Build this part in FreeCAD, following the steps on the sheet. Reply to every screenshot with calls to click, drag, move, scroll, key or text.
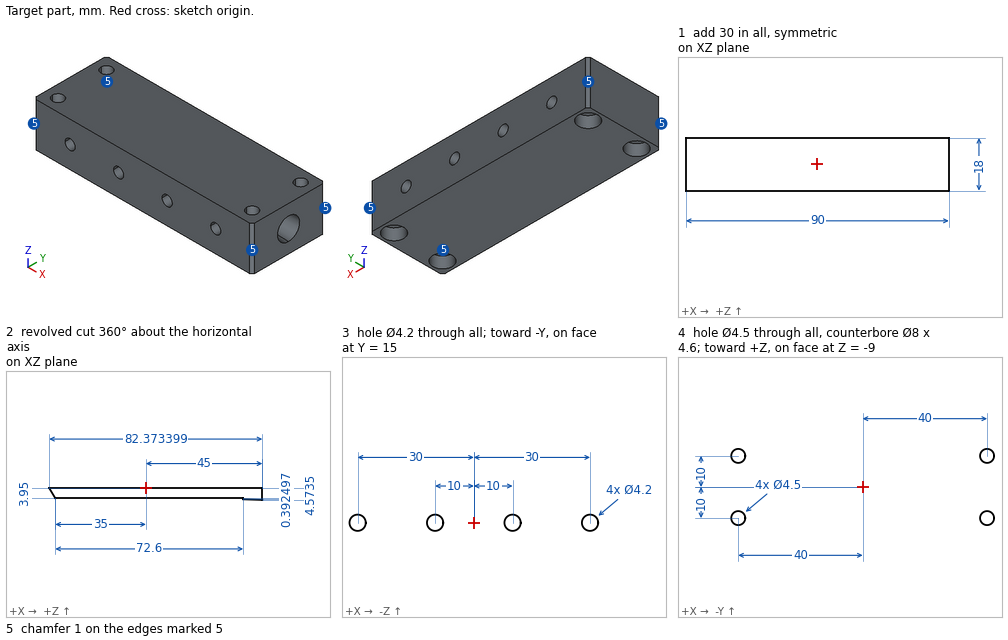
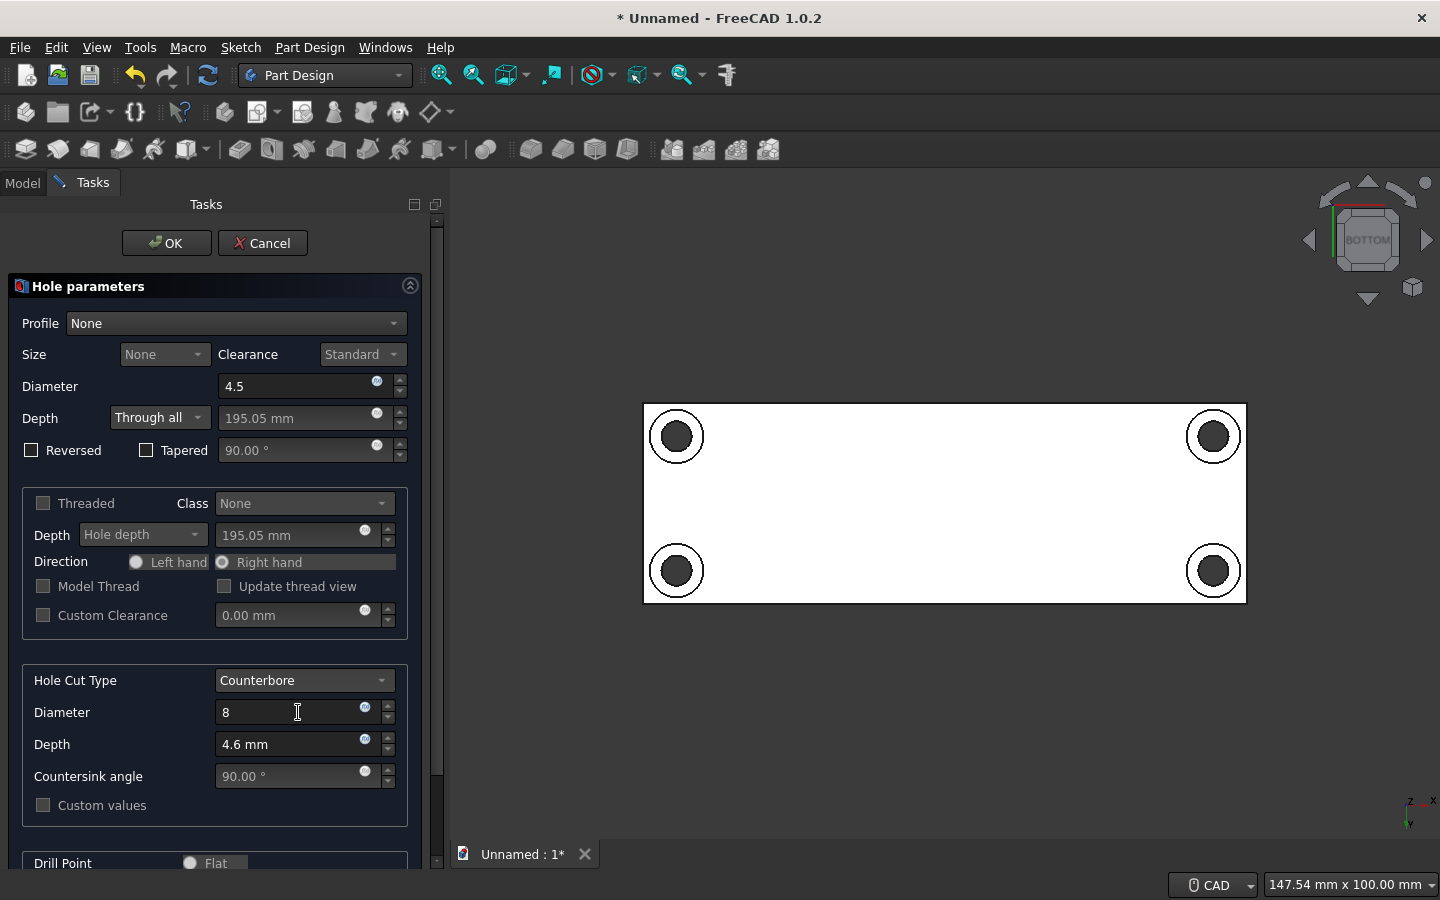
click(167, 243)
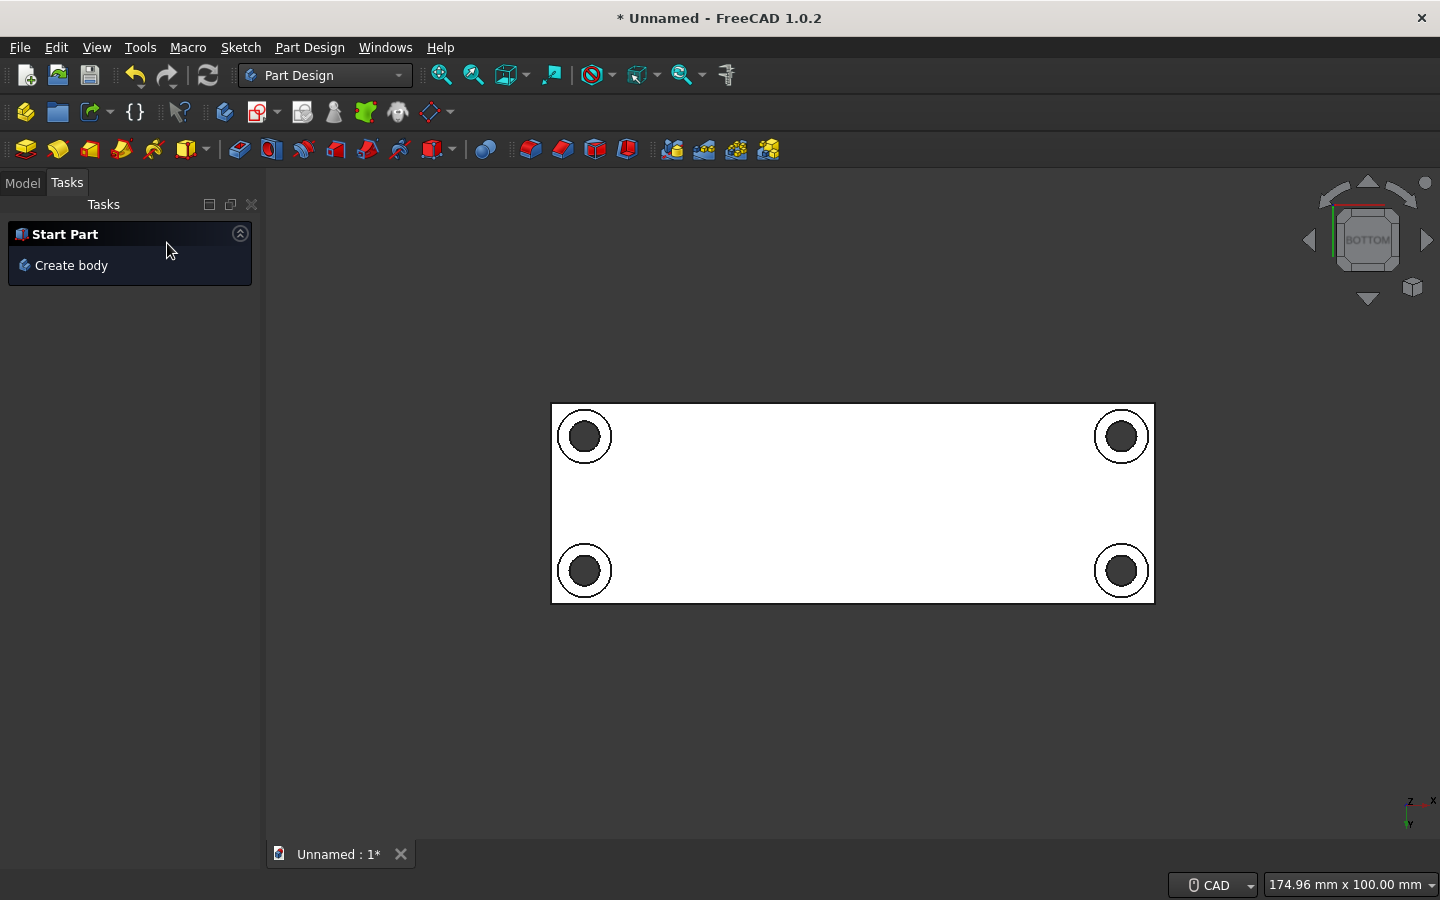
key(0)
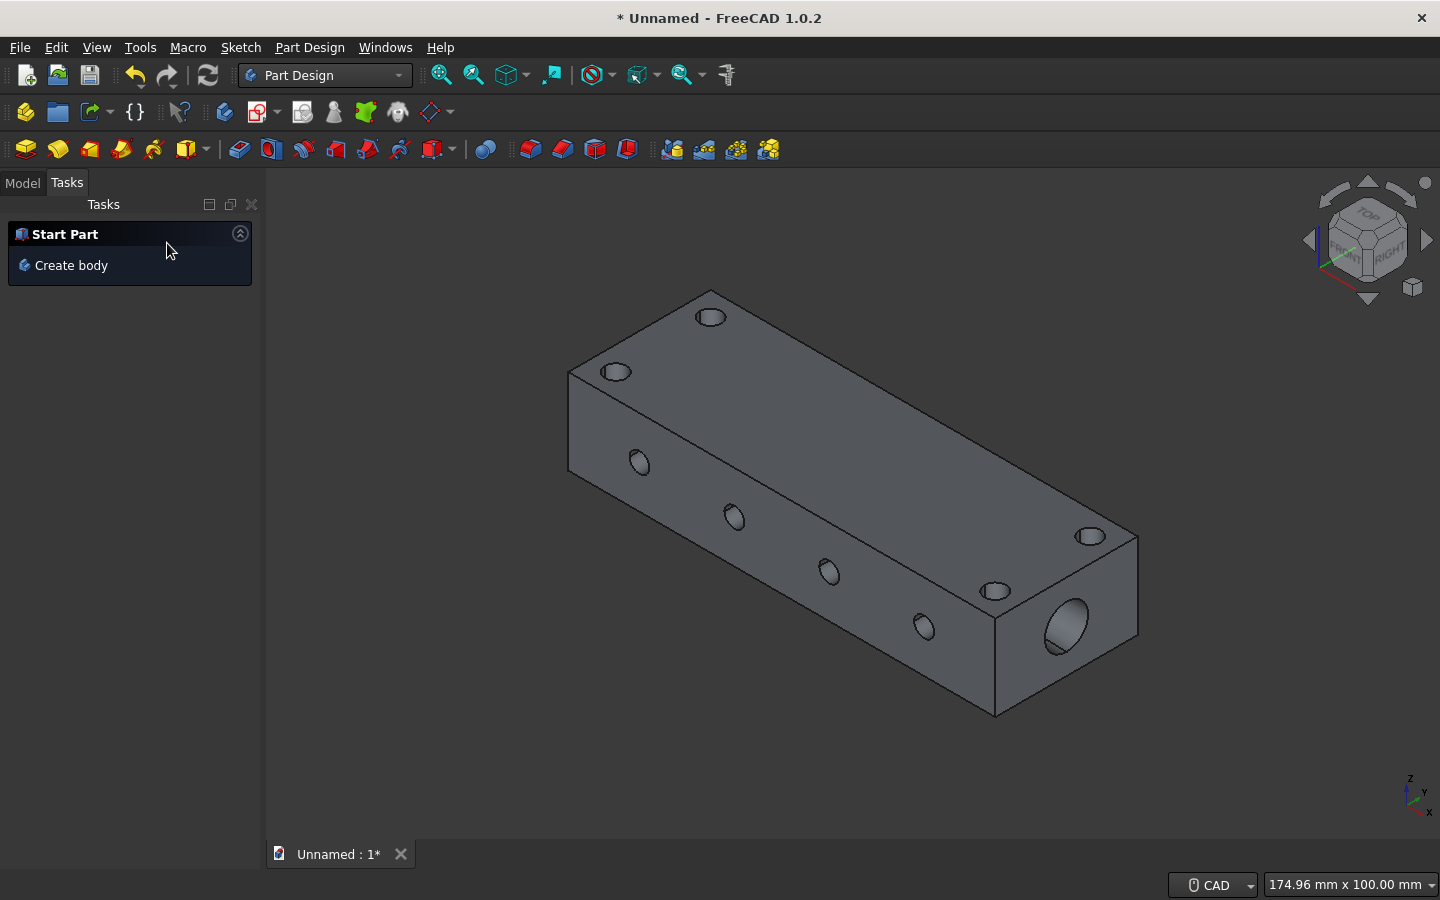
click(995, 667)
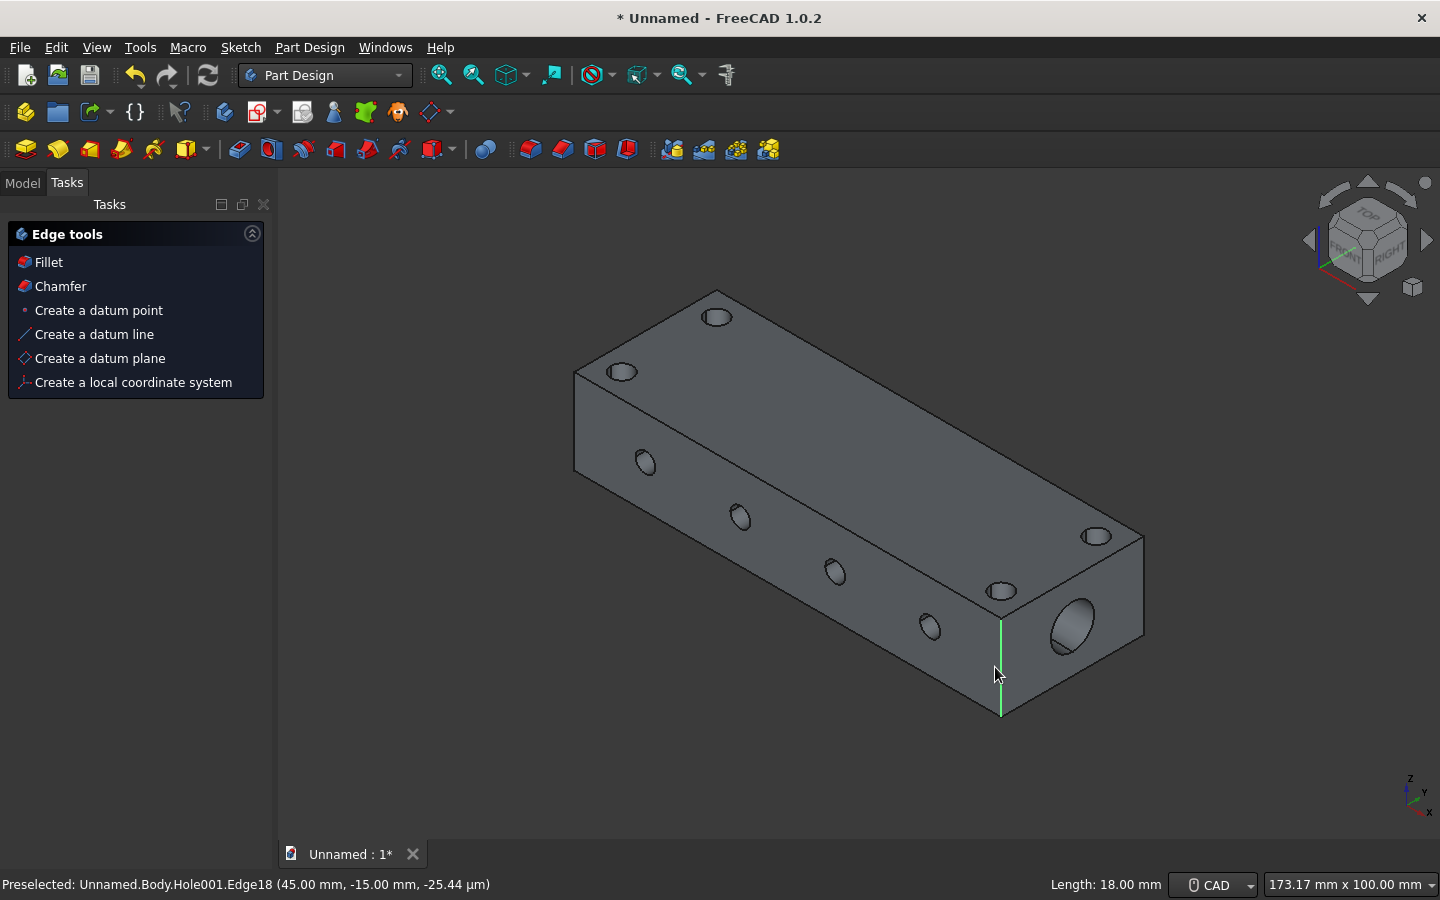
key(2)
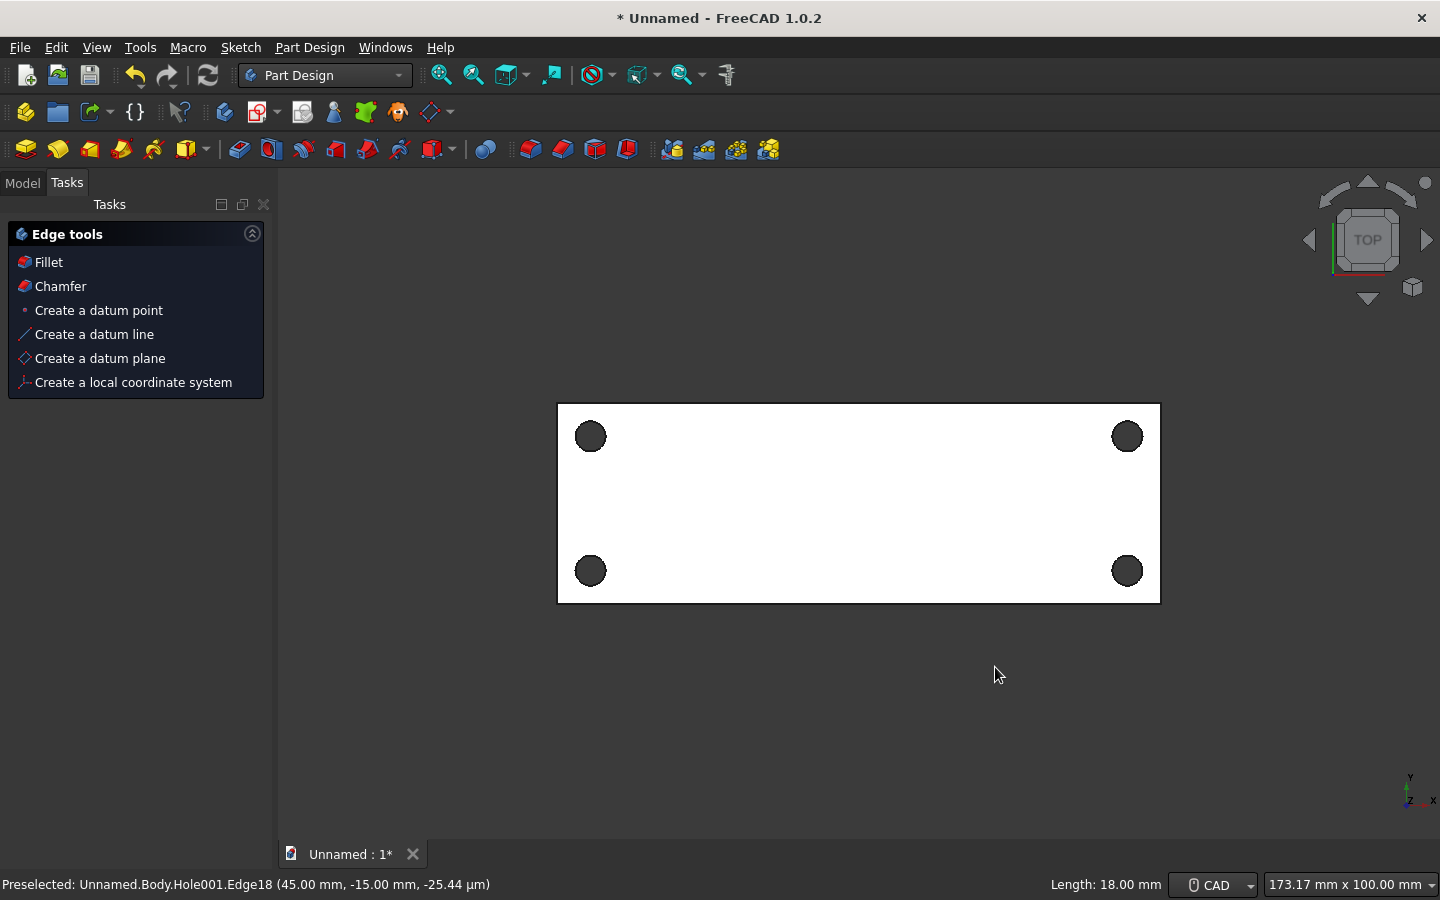
key(1)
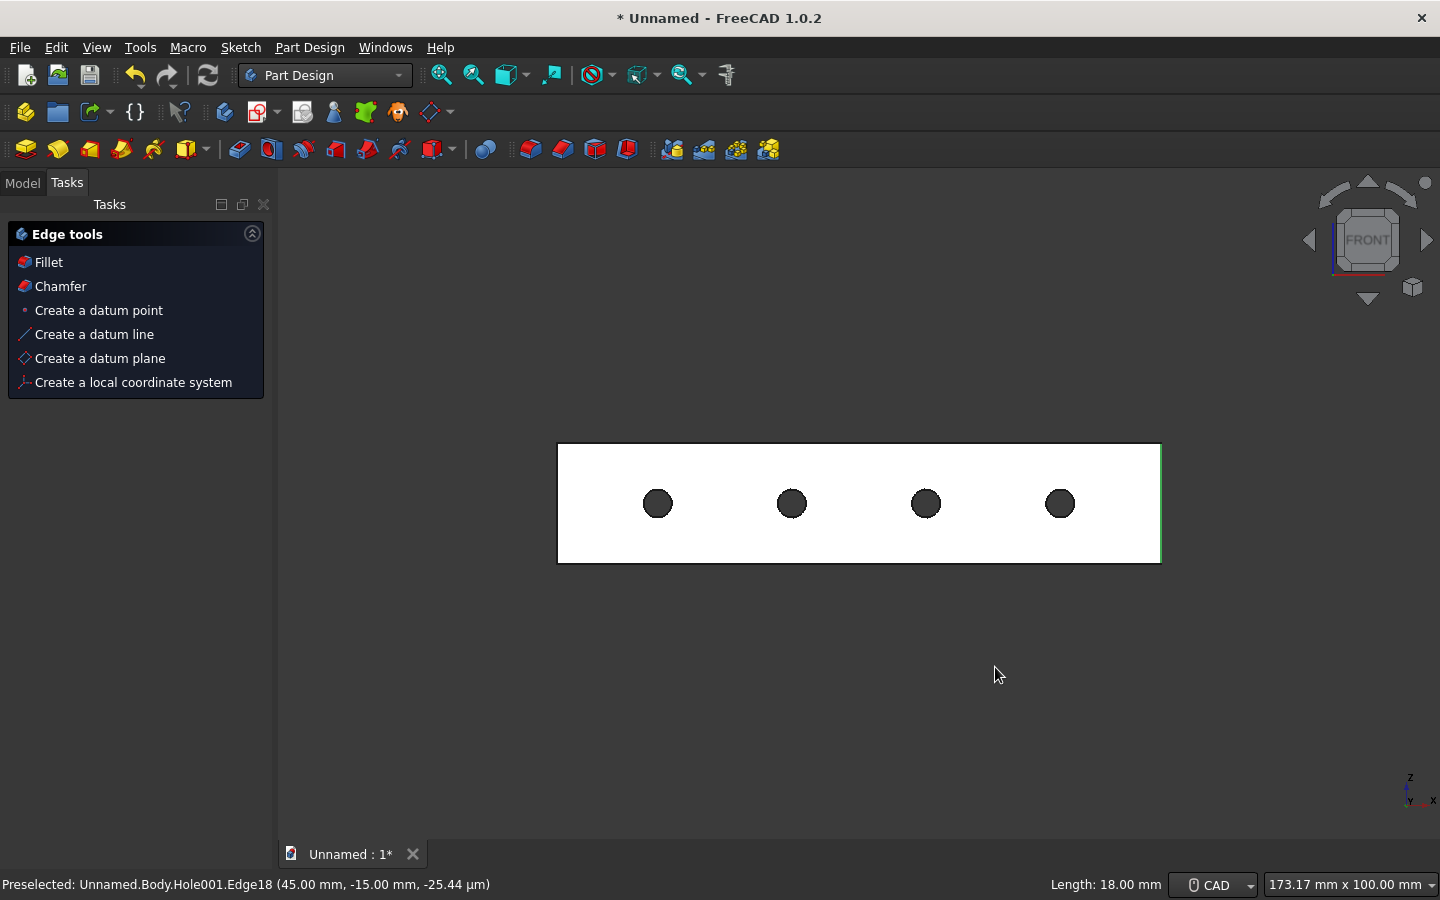
click(557, 503, ctrl)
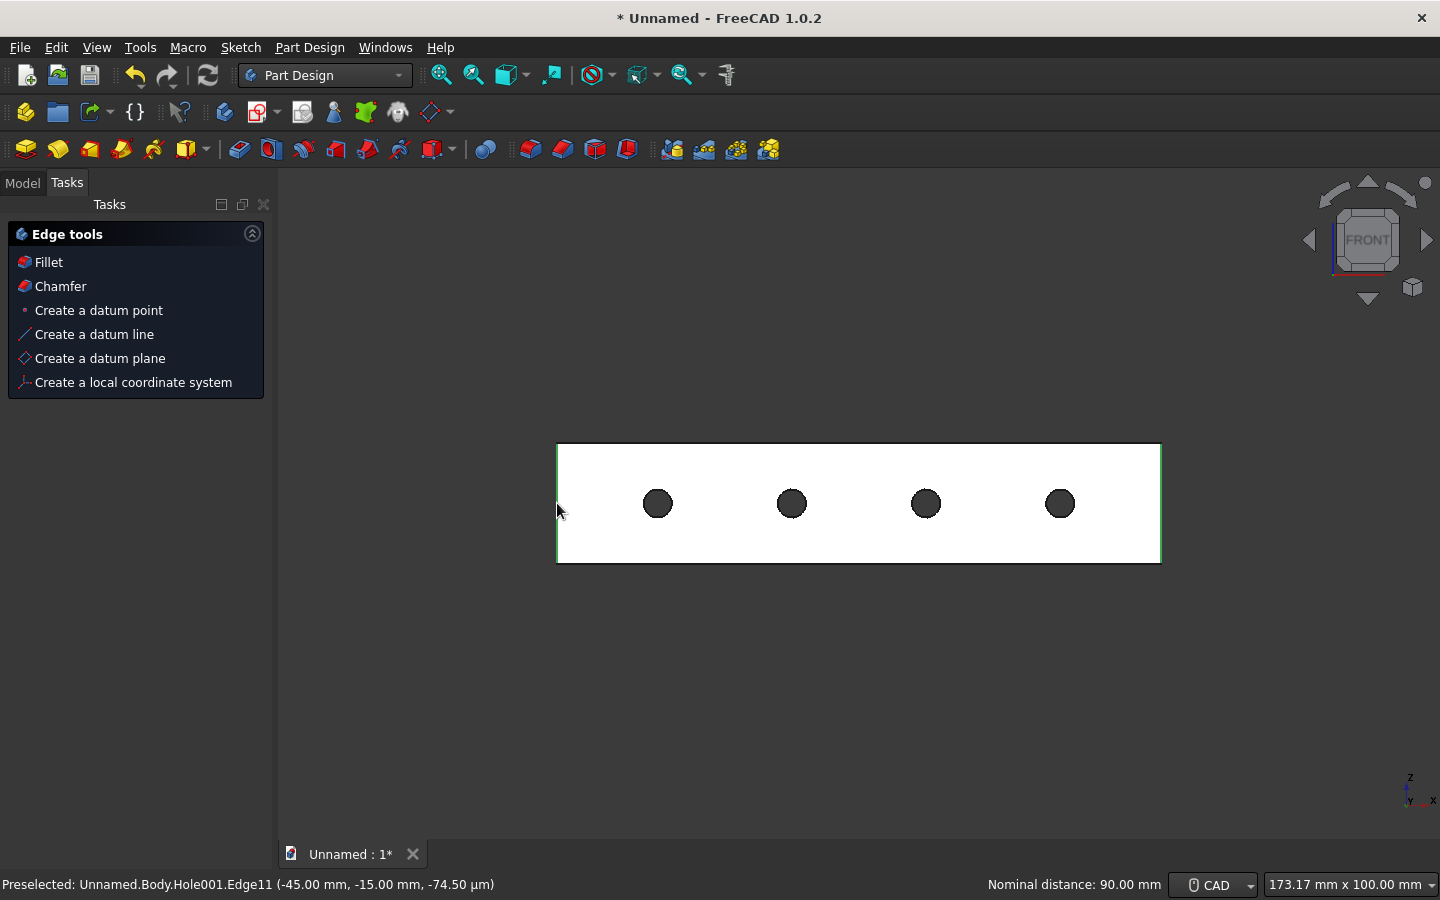
key(3)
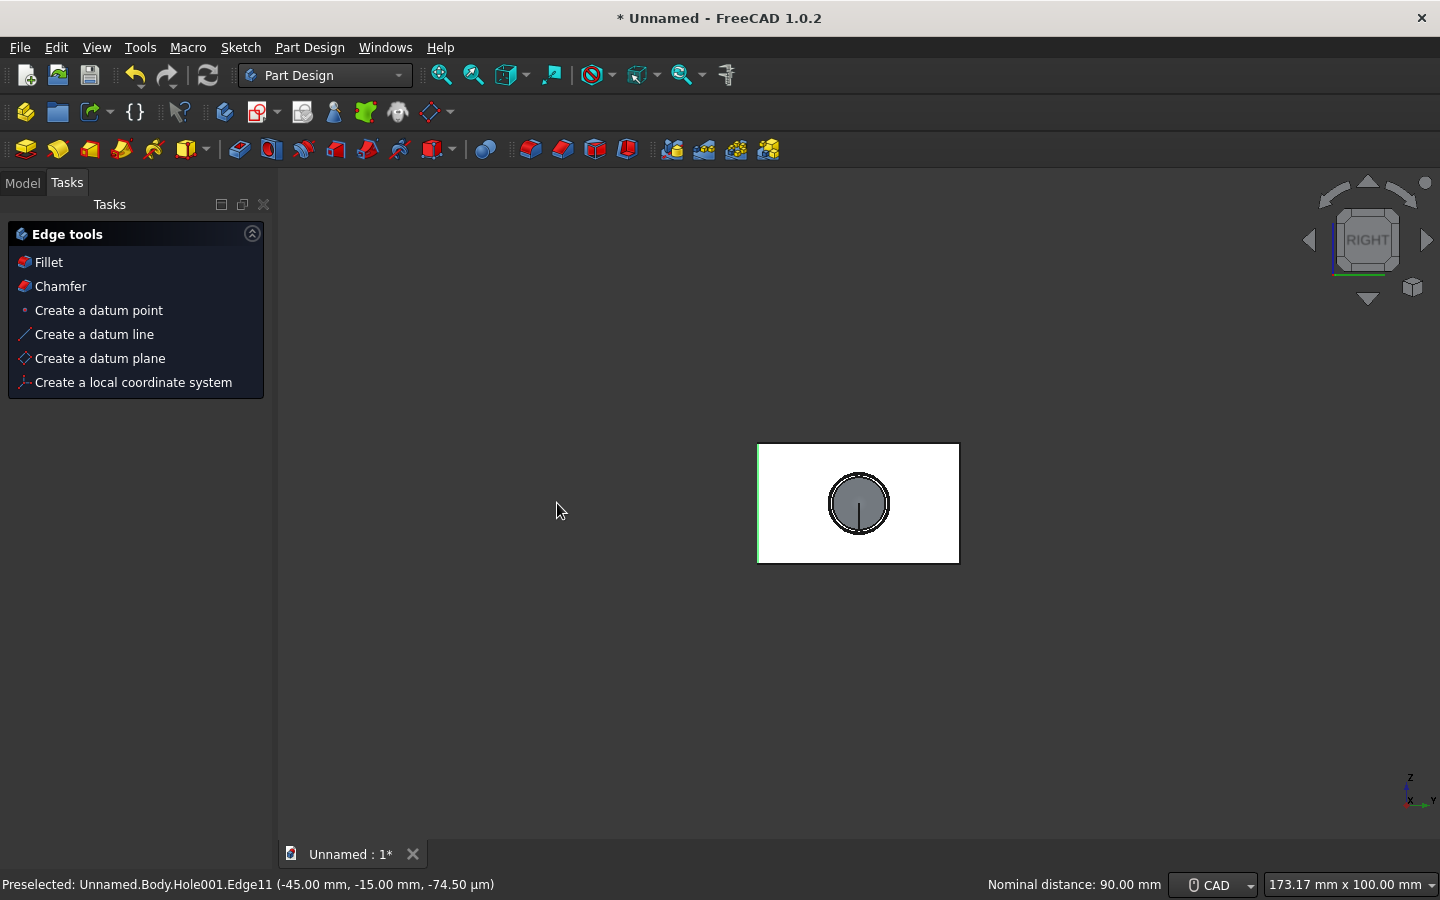
click(442, 76)